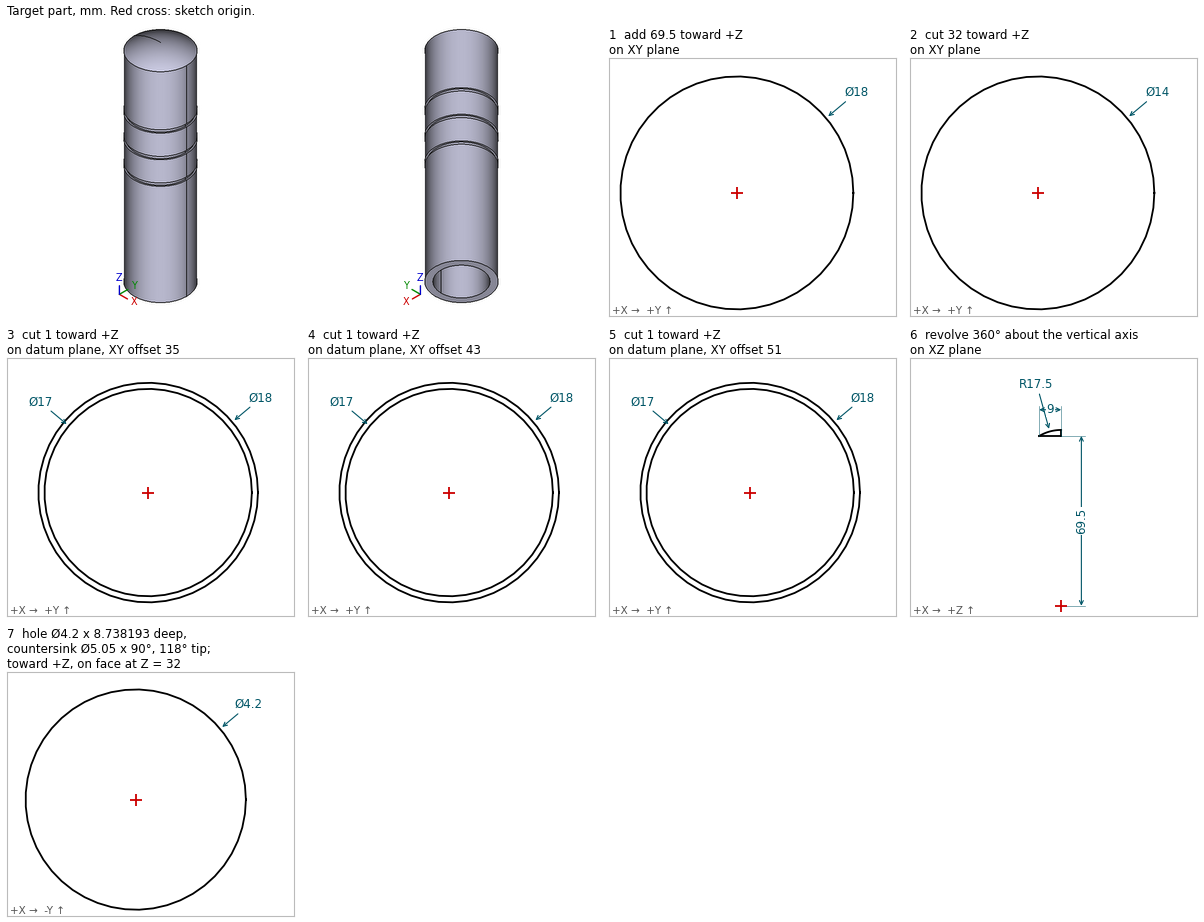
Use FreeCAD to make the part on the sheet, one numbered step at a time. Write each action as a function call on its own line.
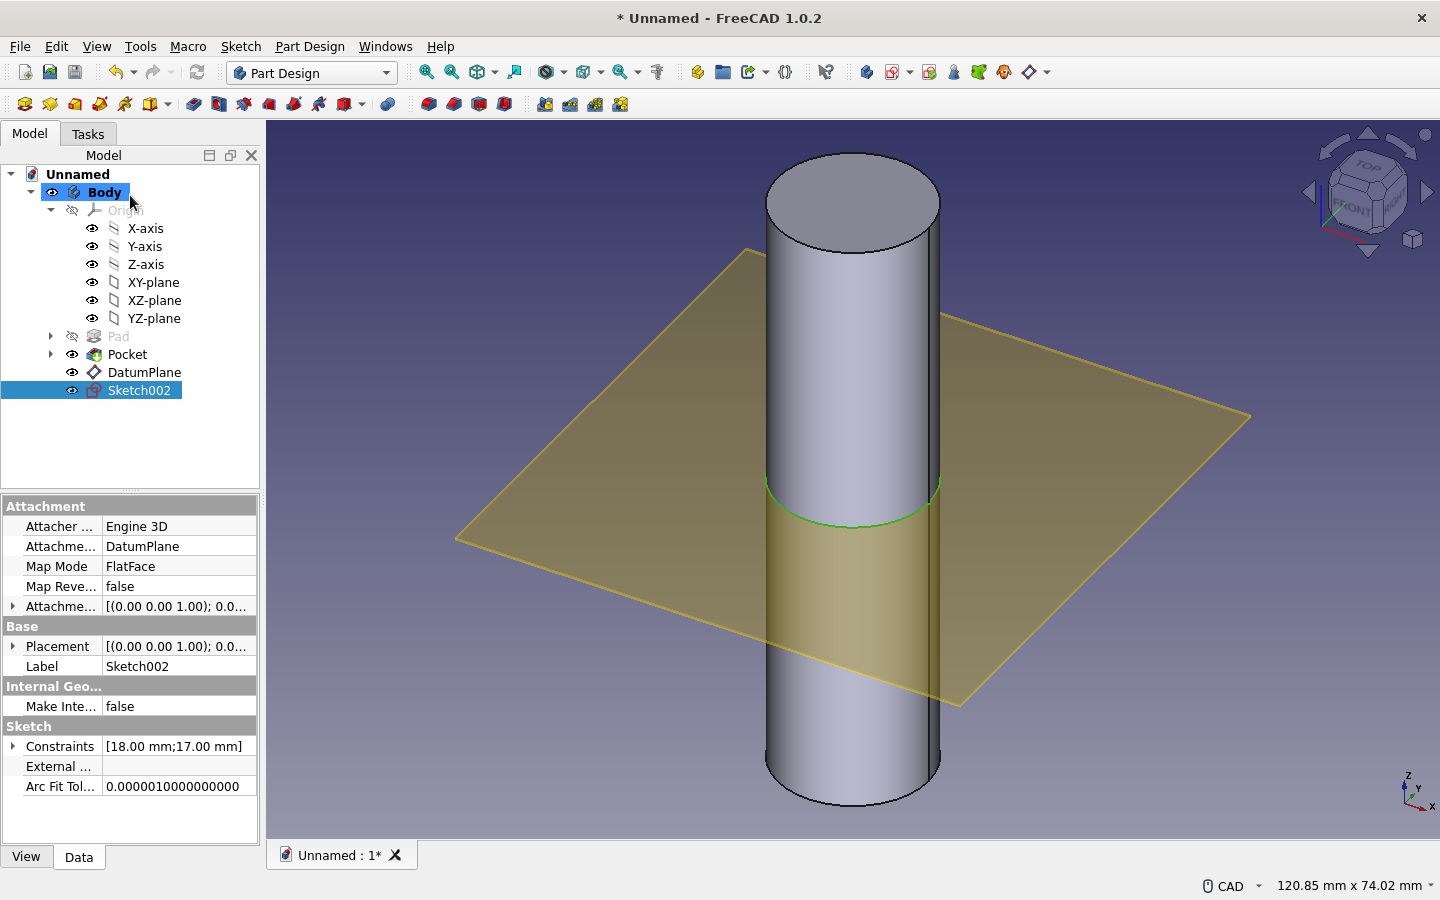
click(194, 104)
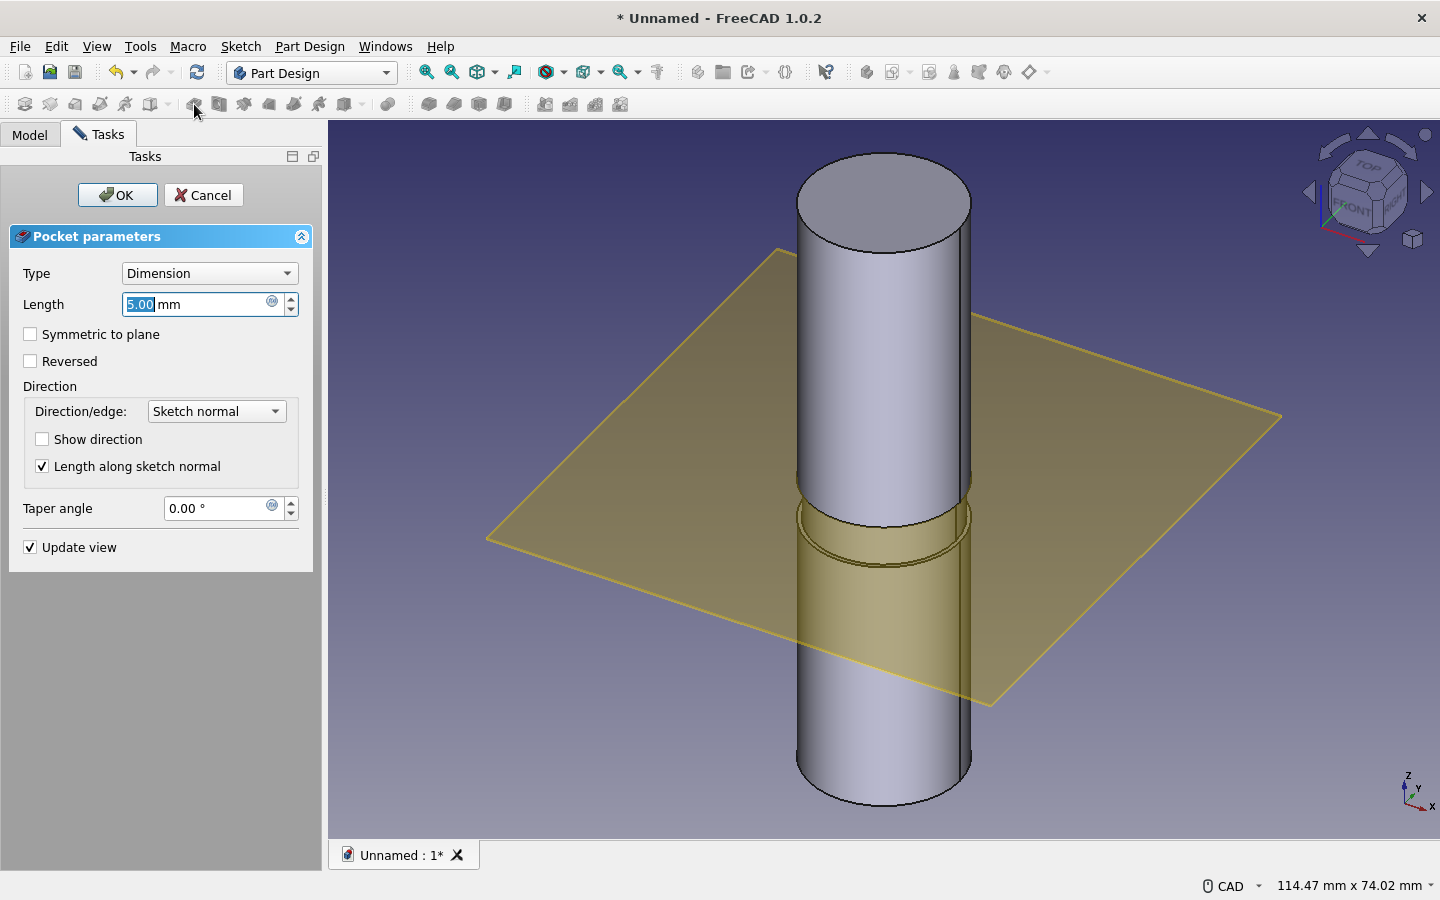
text(1)
key(Tab)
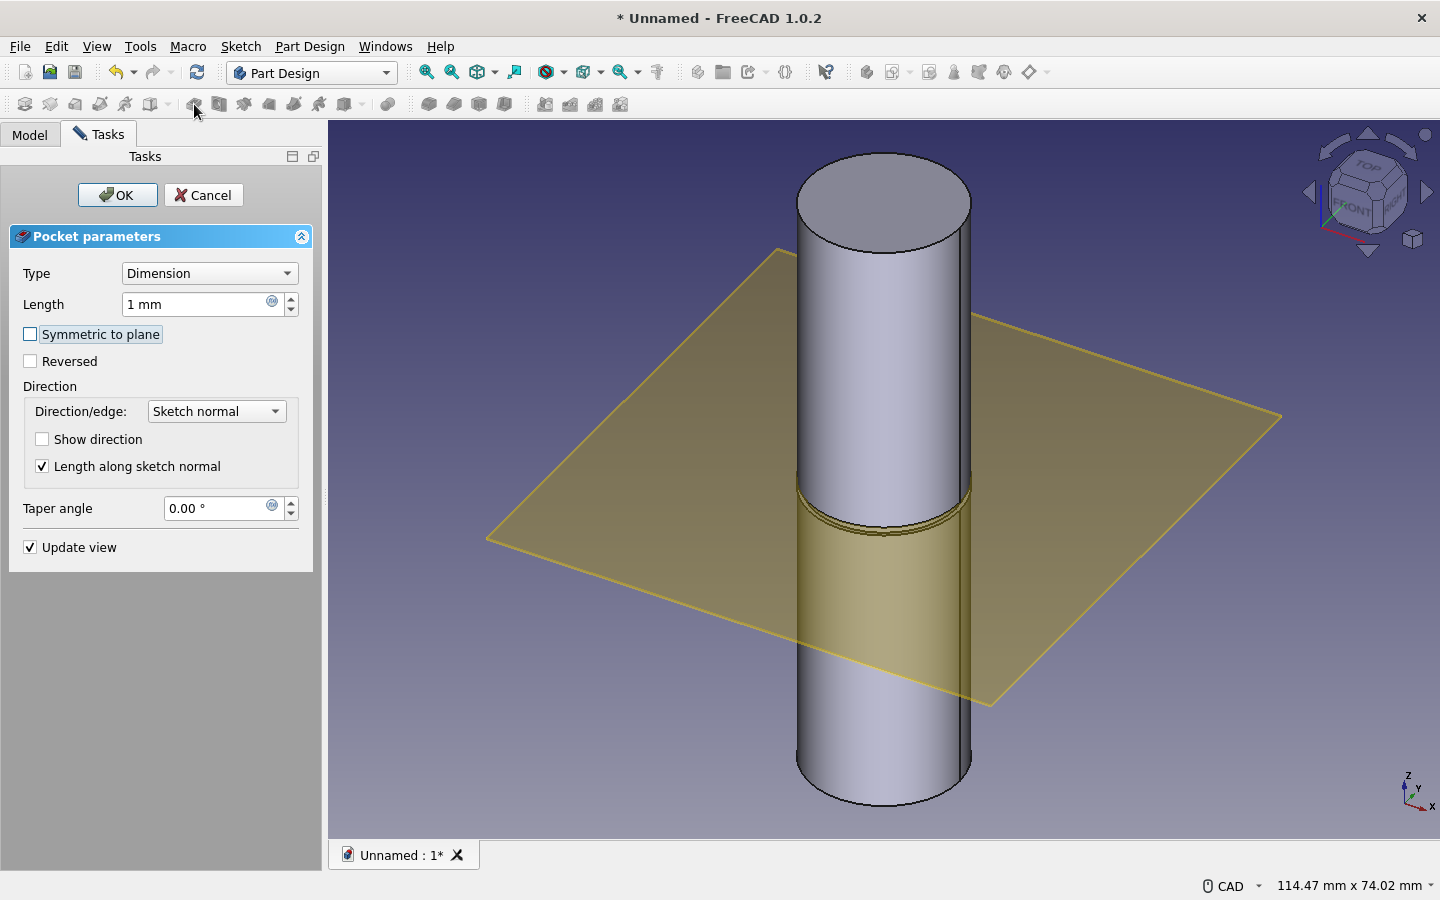
click(31, 361)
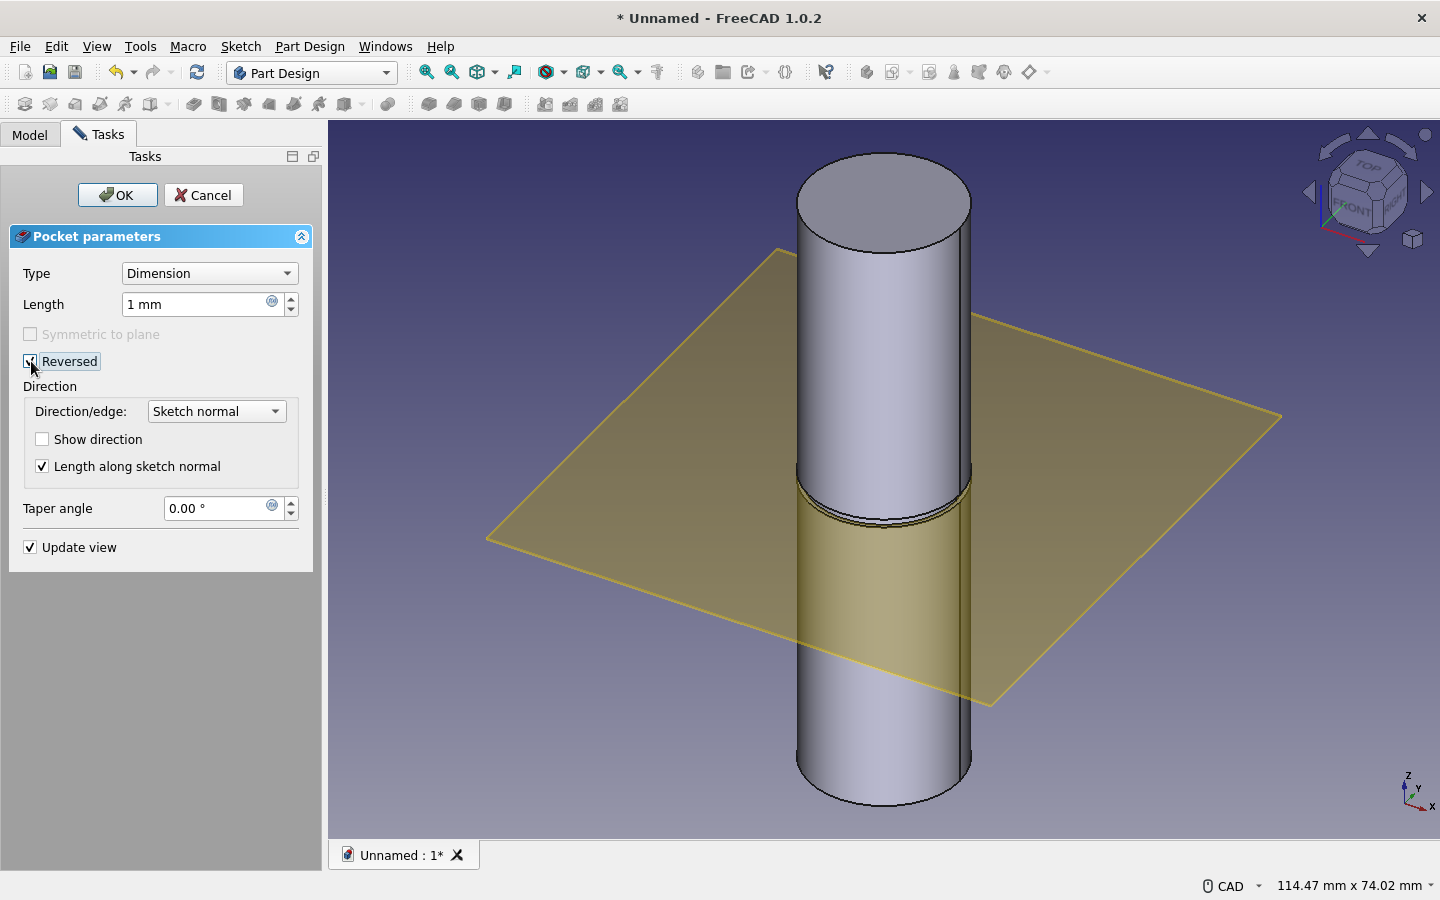
click(118, 195)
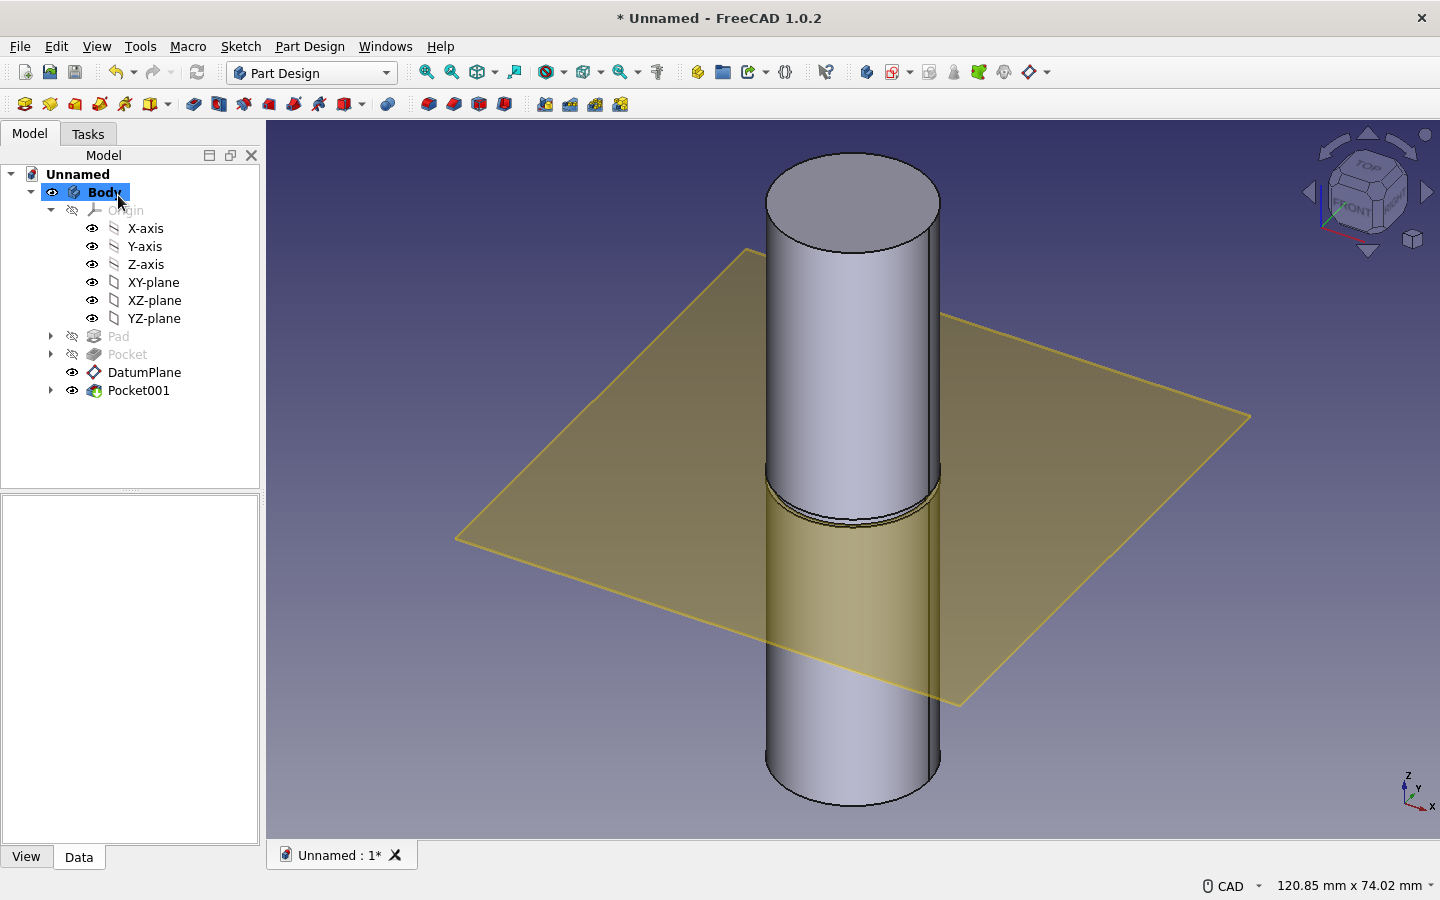
click(117, 372)
key(space)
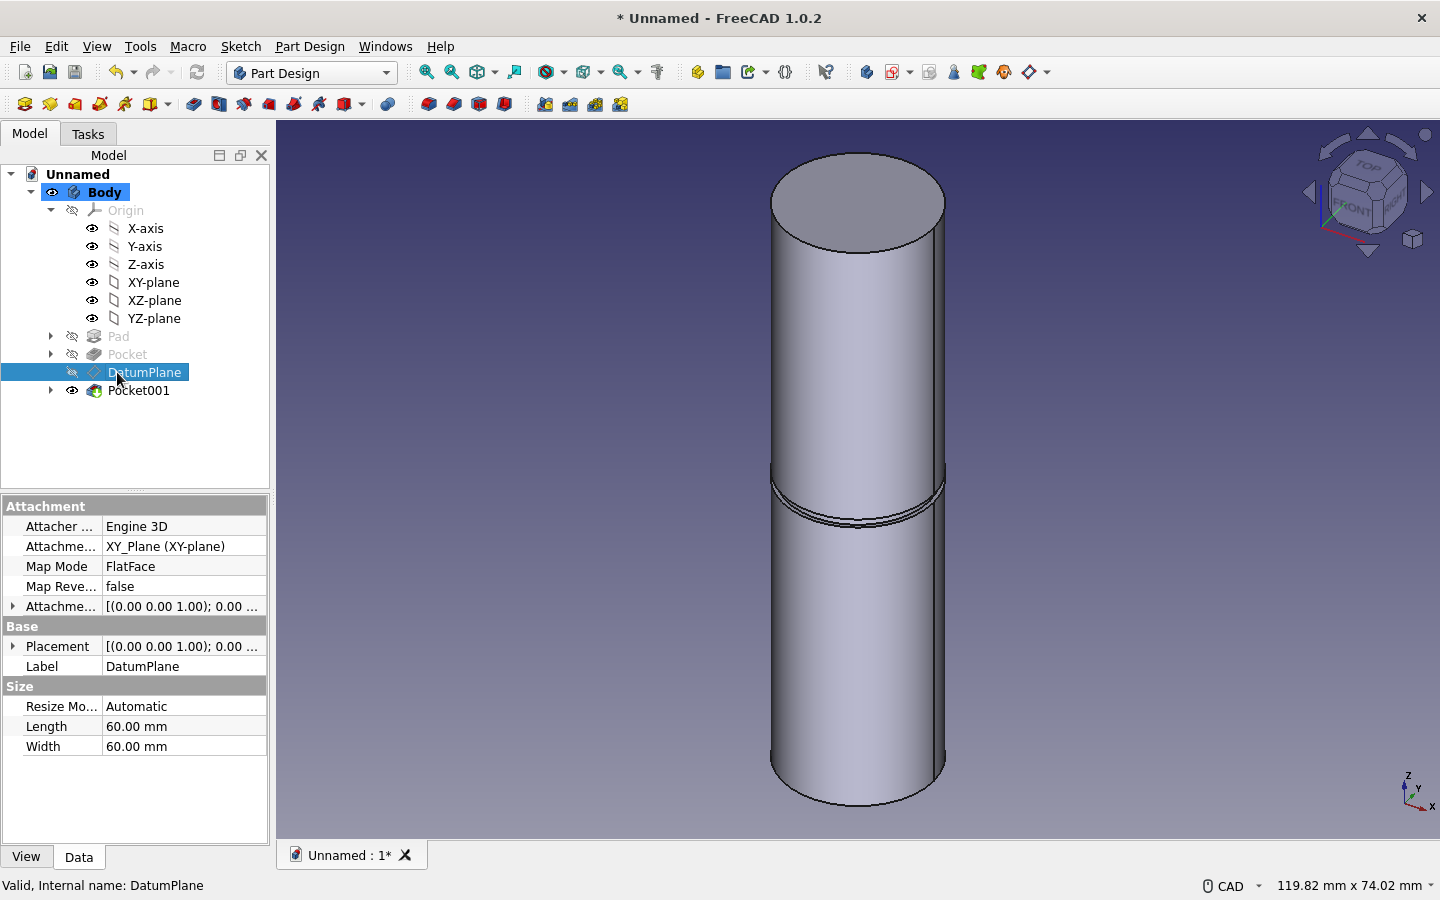
click(137, 282)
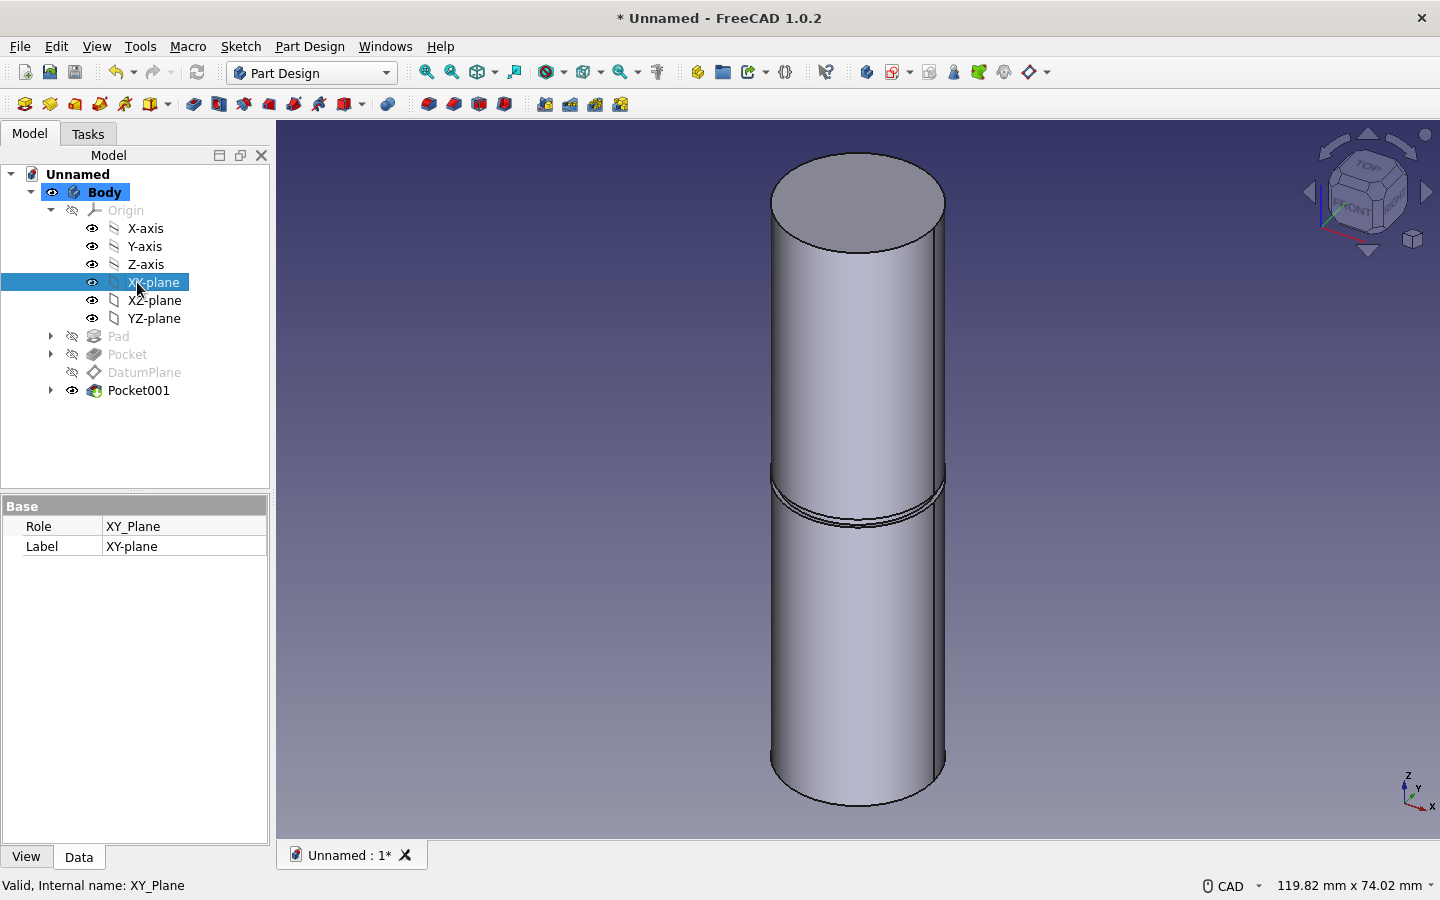
click(1028, 72)